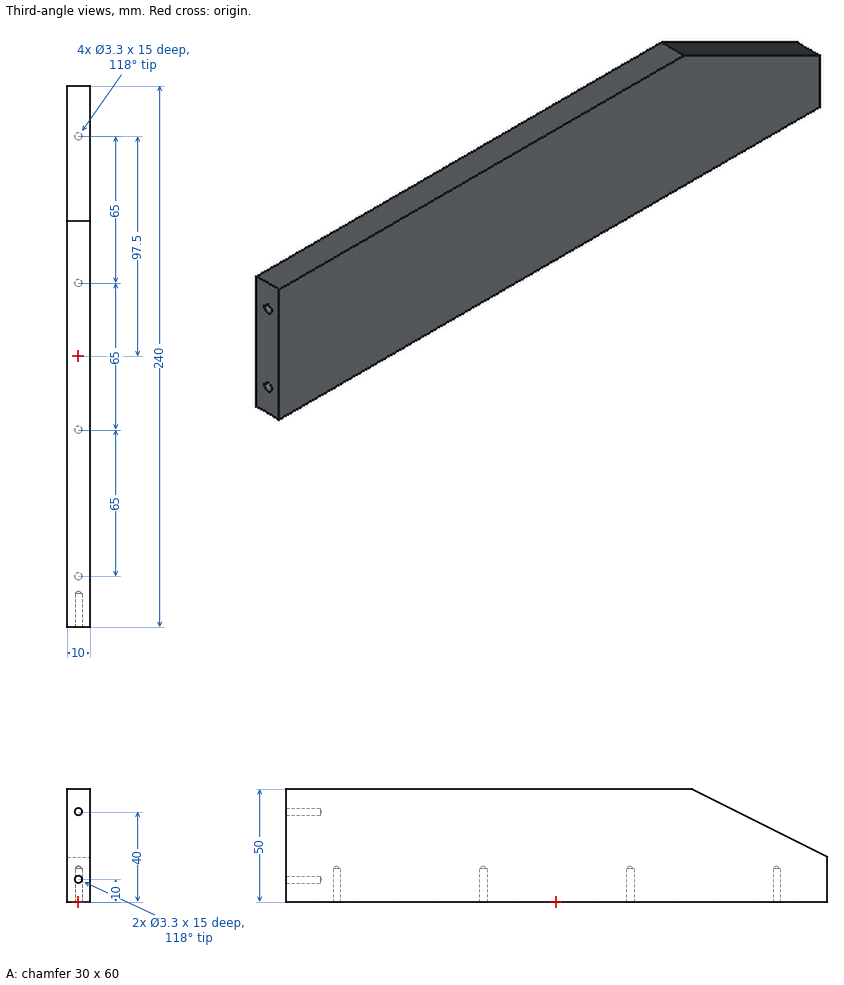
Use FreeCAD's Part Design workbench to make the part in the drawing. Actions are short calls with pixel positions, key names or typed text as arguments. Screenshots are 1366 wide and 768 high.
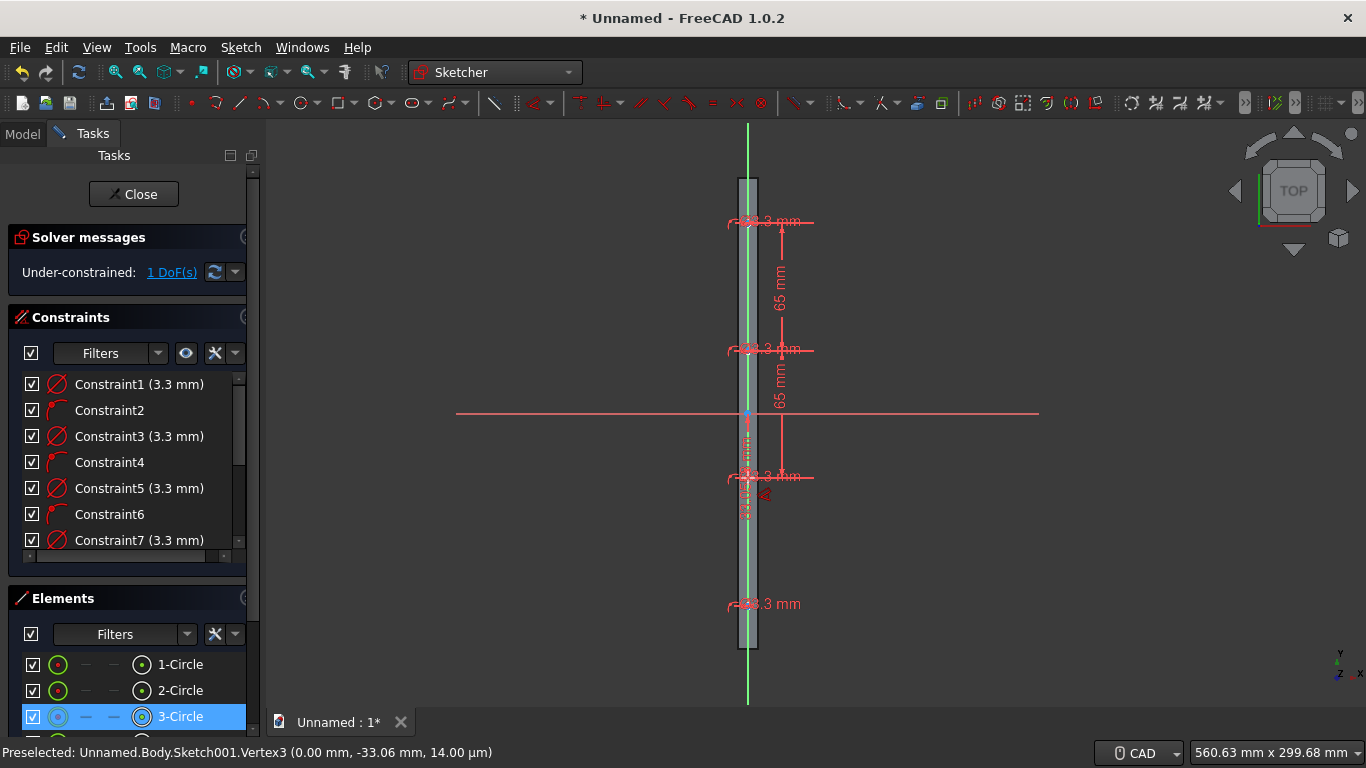
click(748, 606)
click(782, 542)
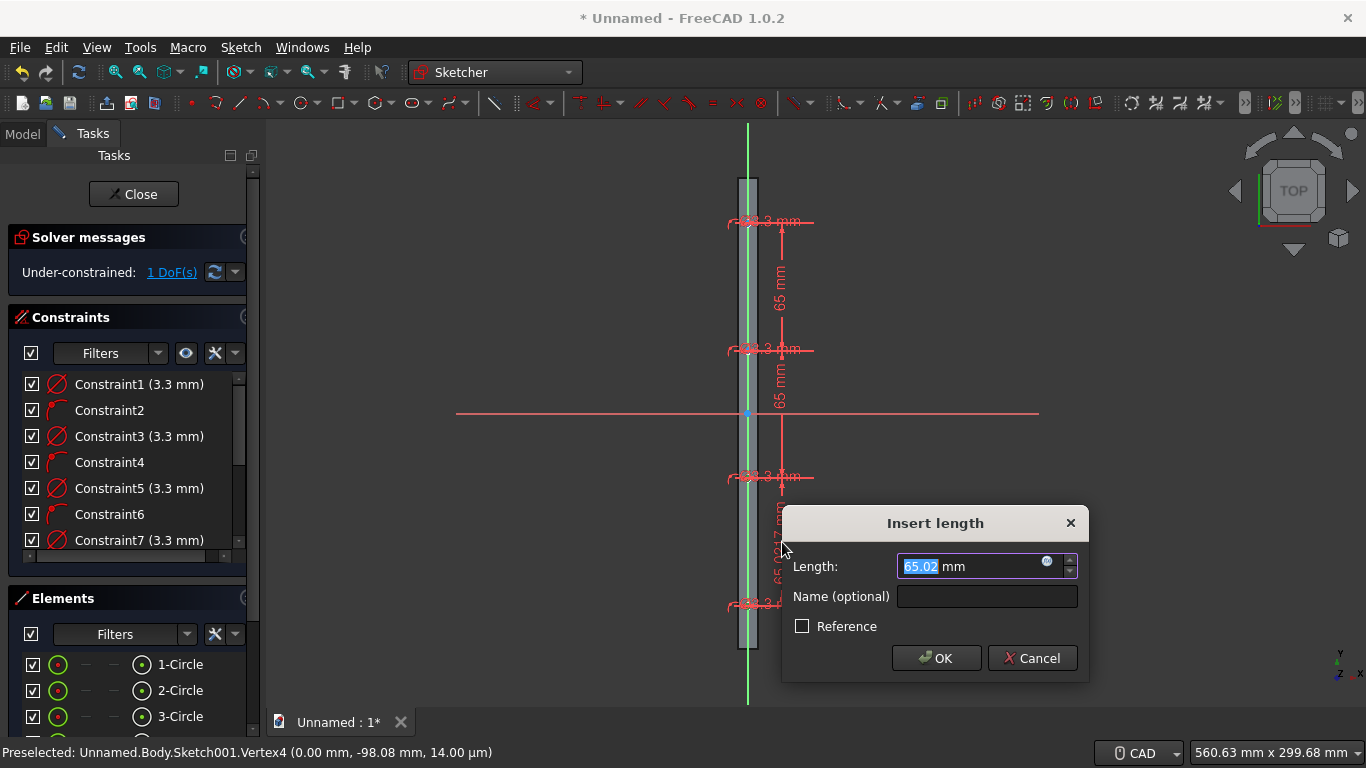
text(65)
key(Return)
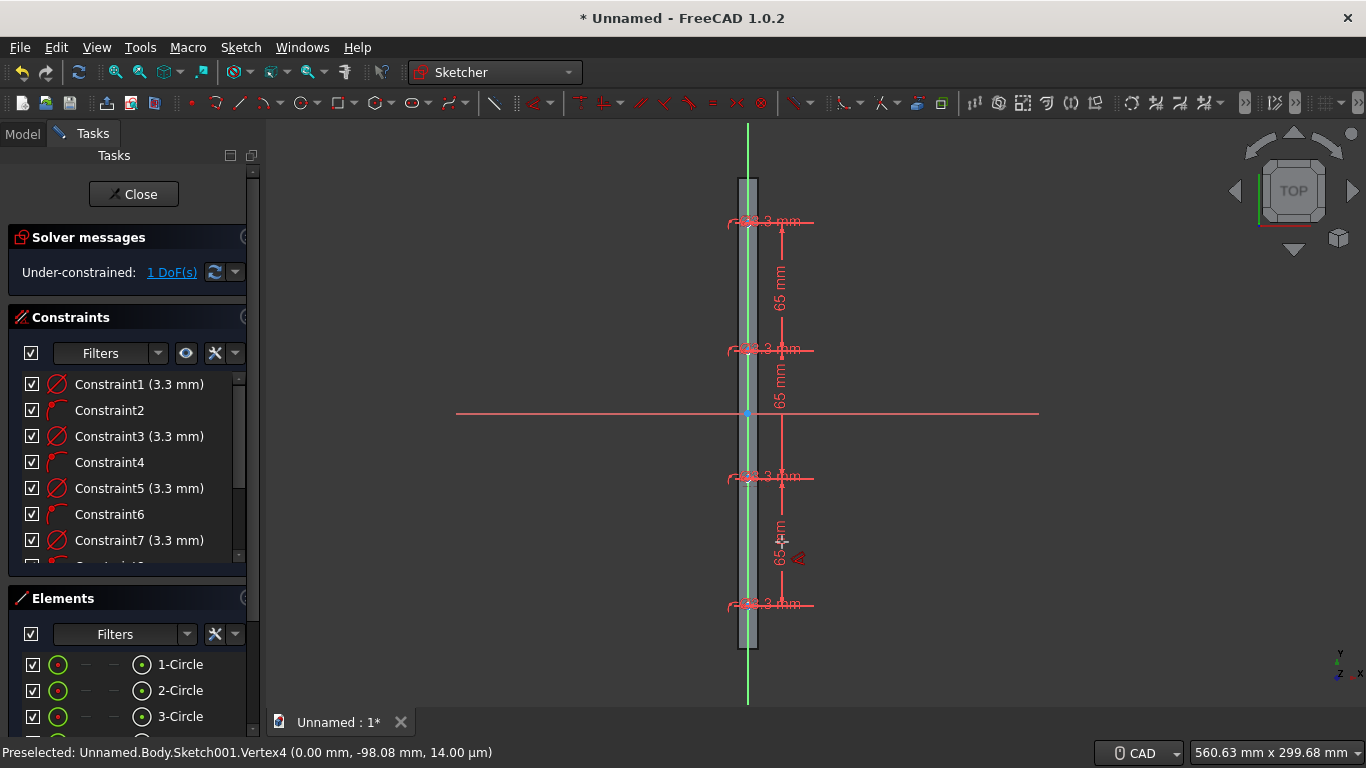
click(748, 223)
click(782, 319)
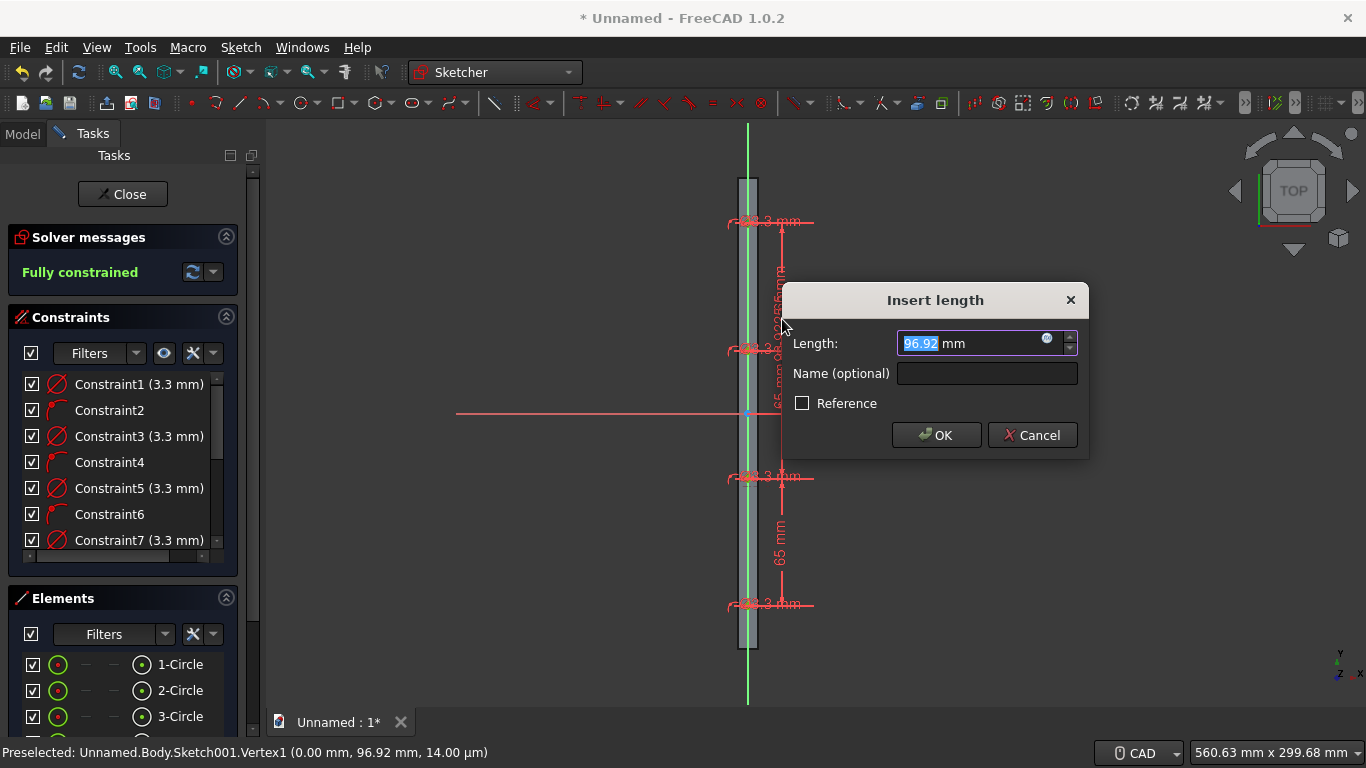
text(97.5)
key(Return)
key(Escape)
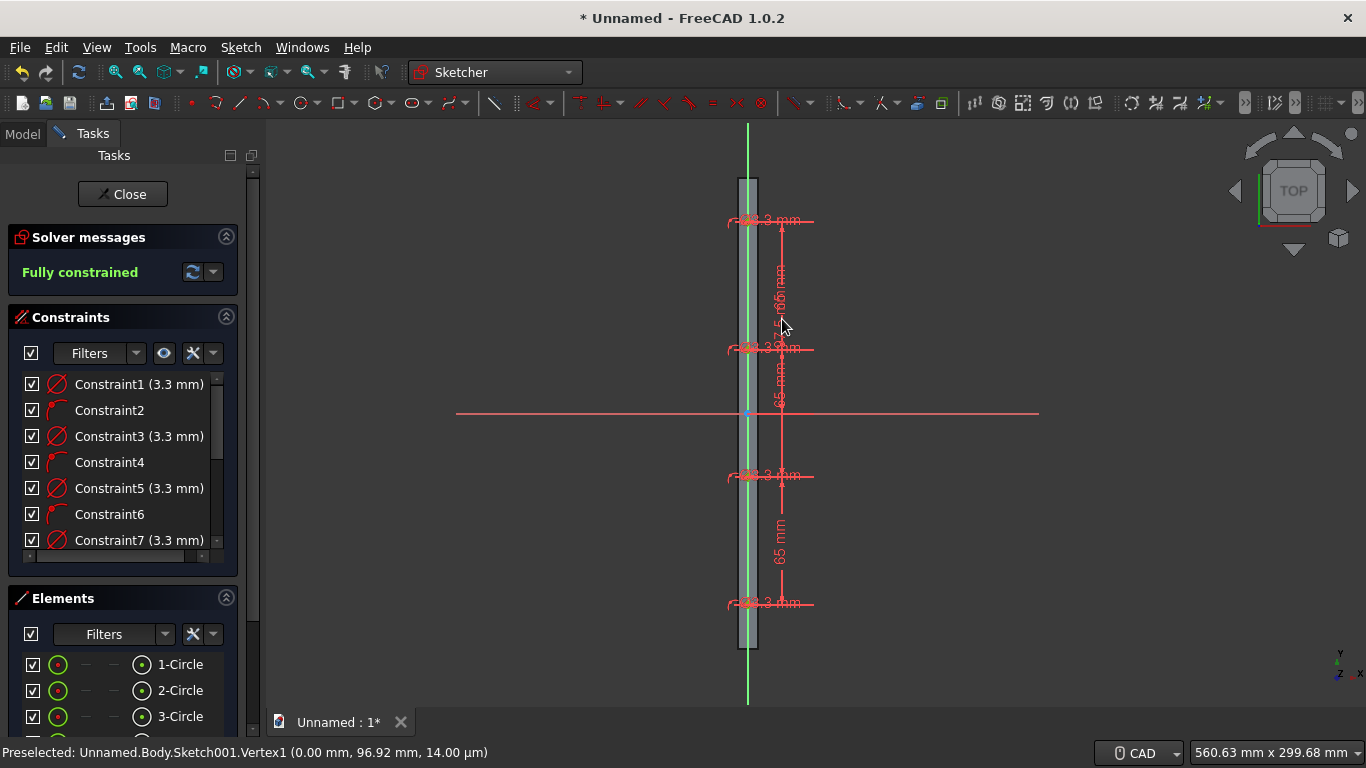
click(123, 194)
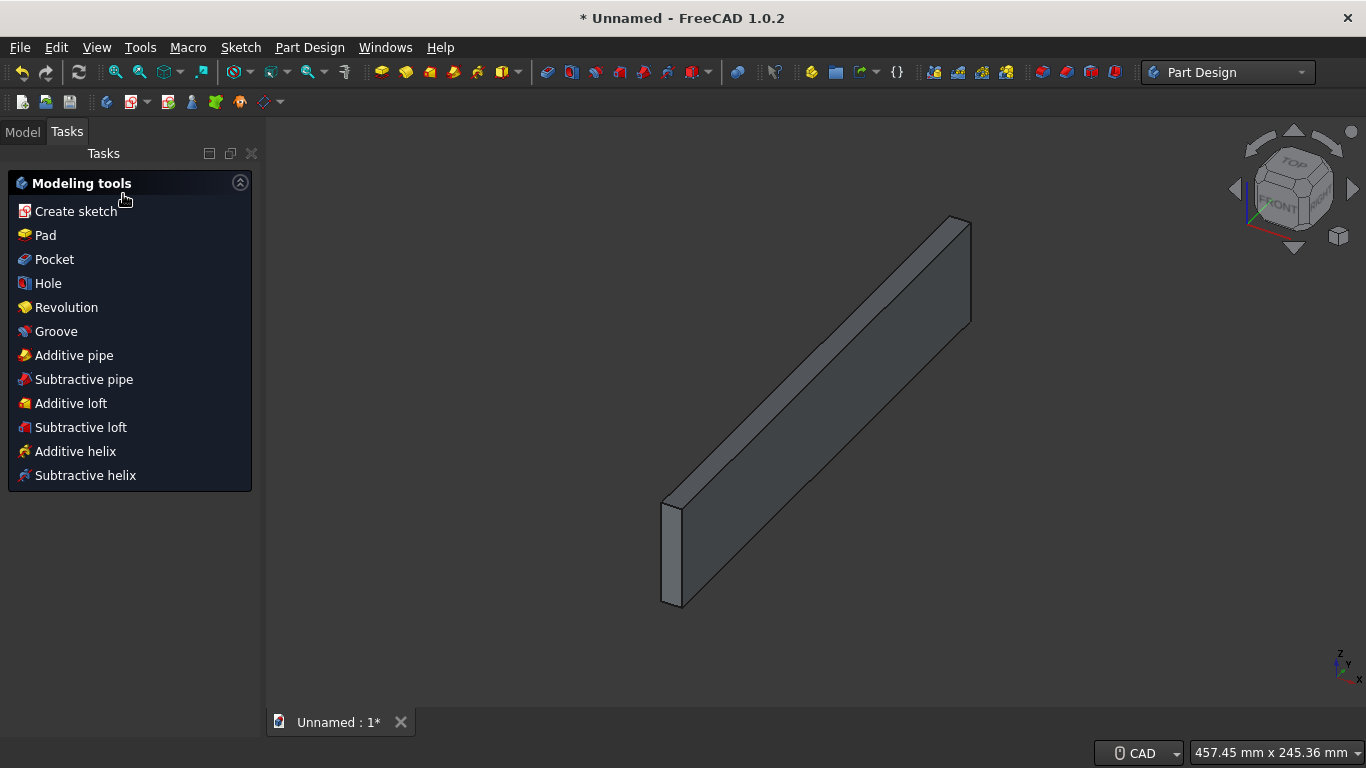
click(572, 72)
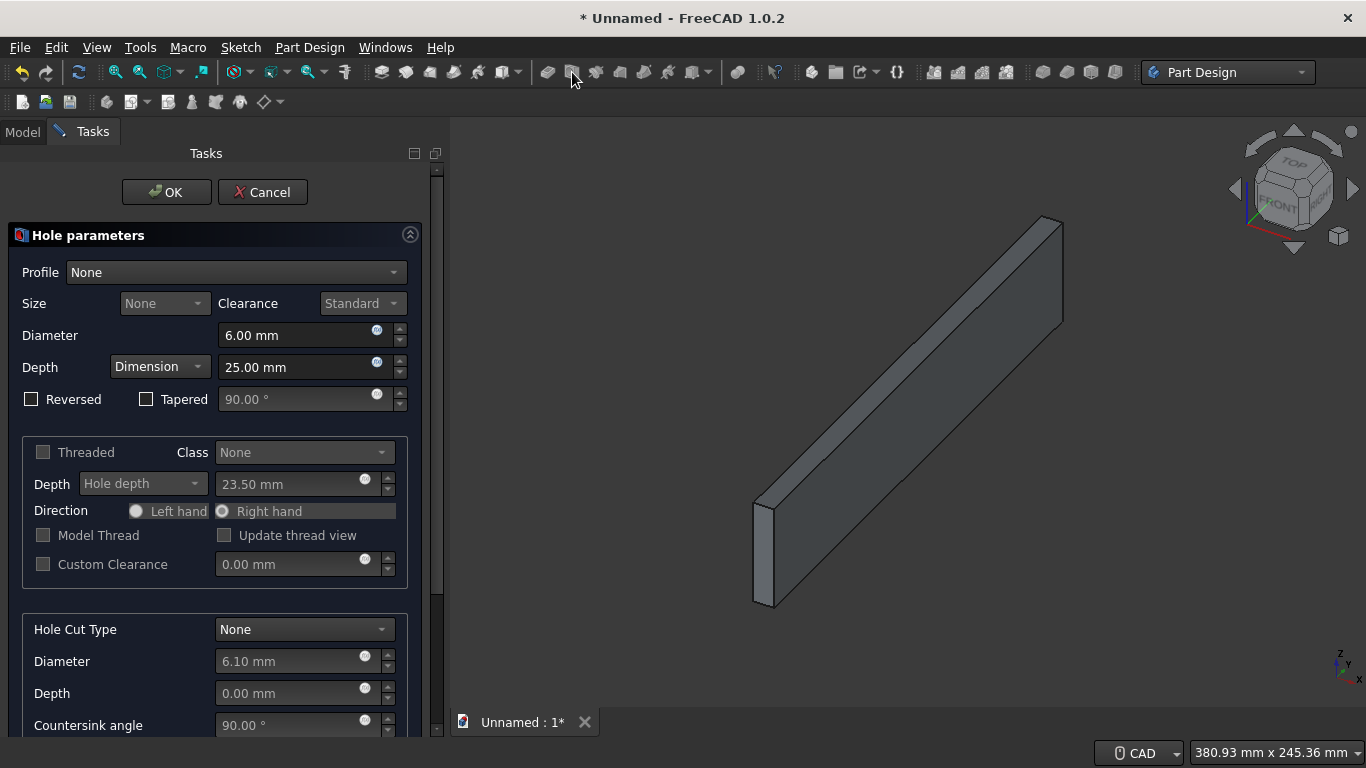
triple_click(305, 335)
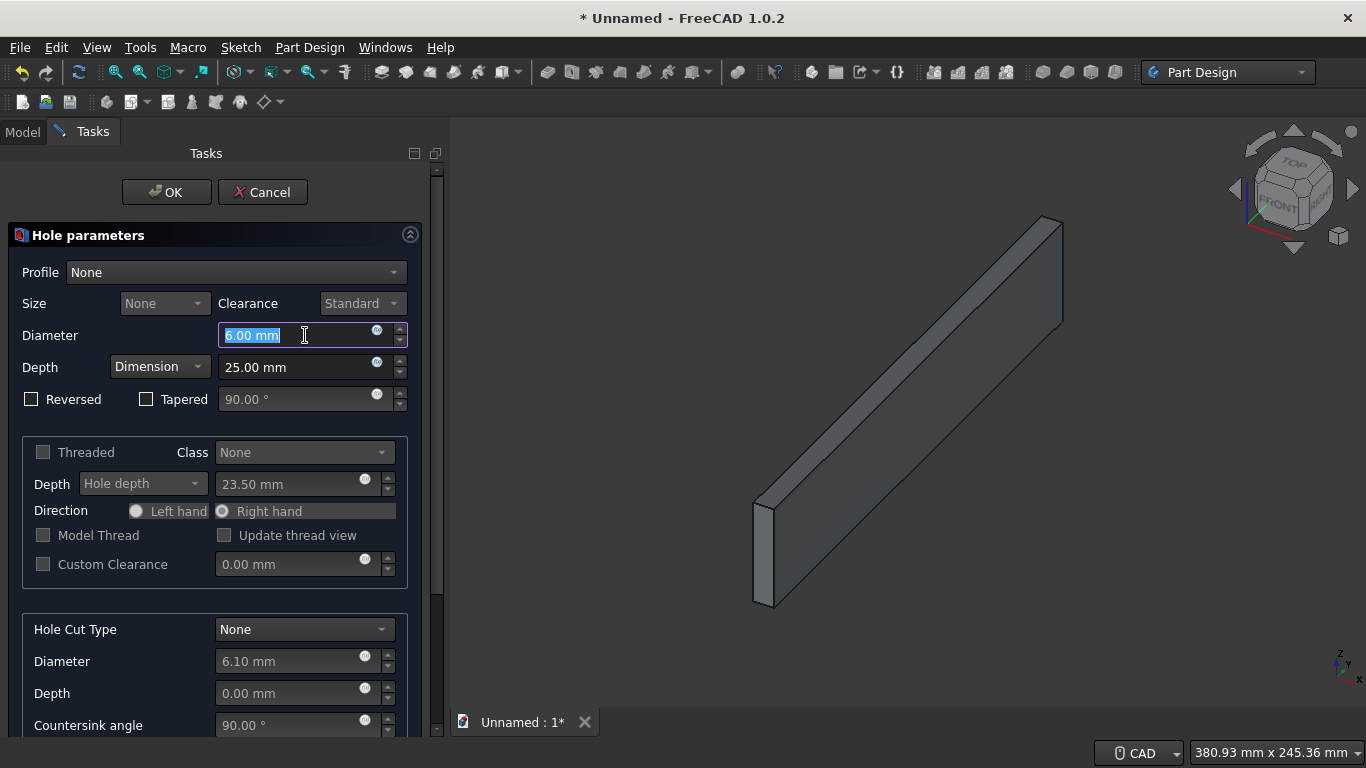
text(3.3)
key(Tab)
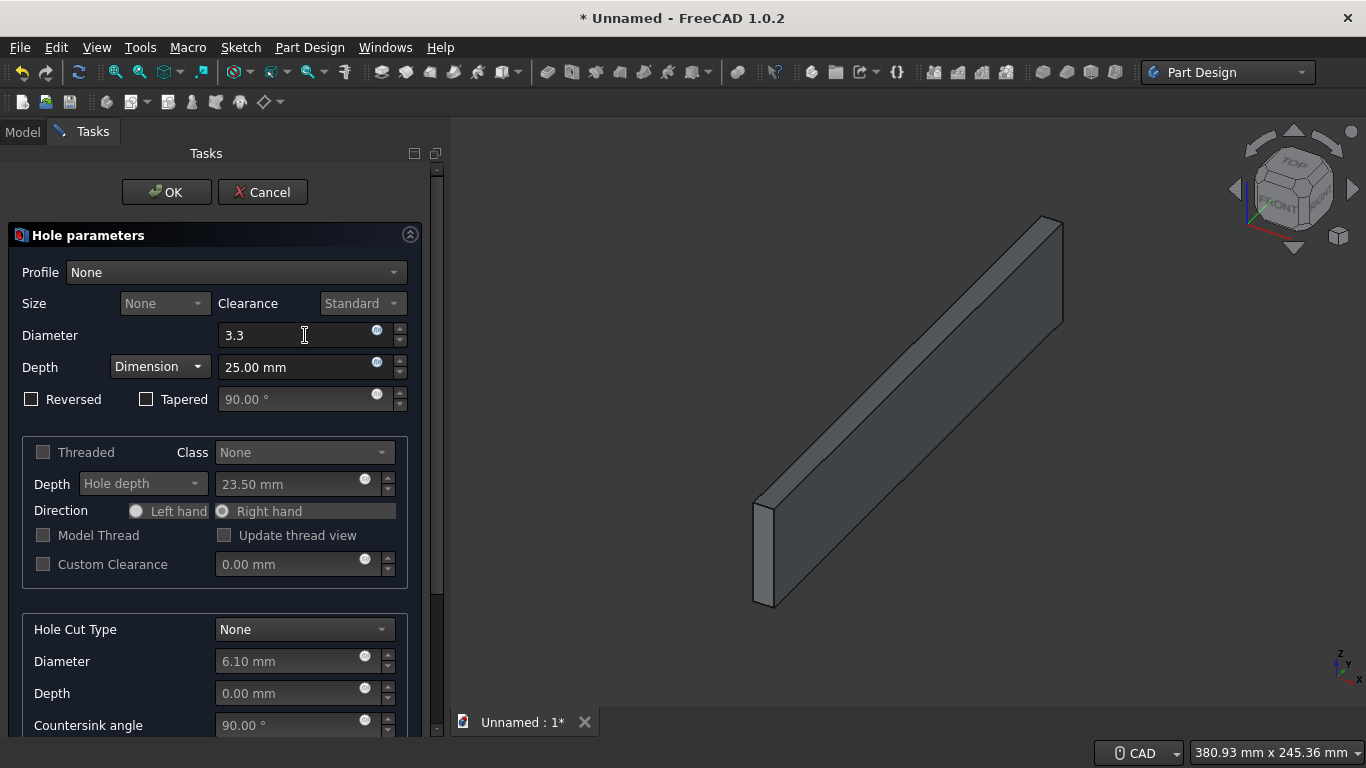
triple_click(305, 367)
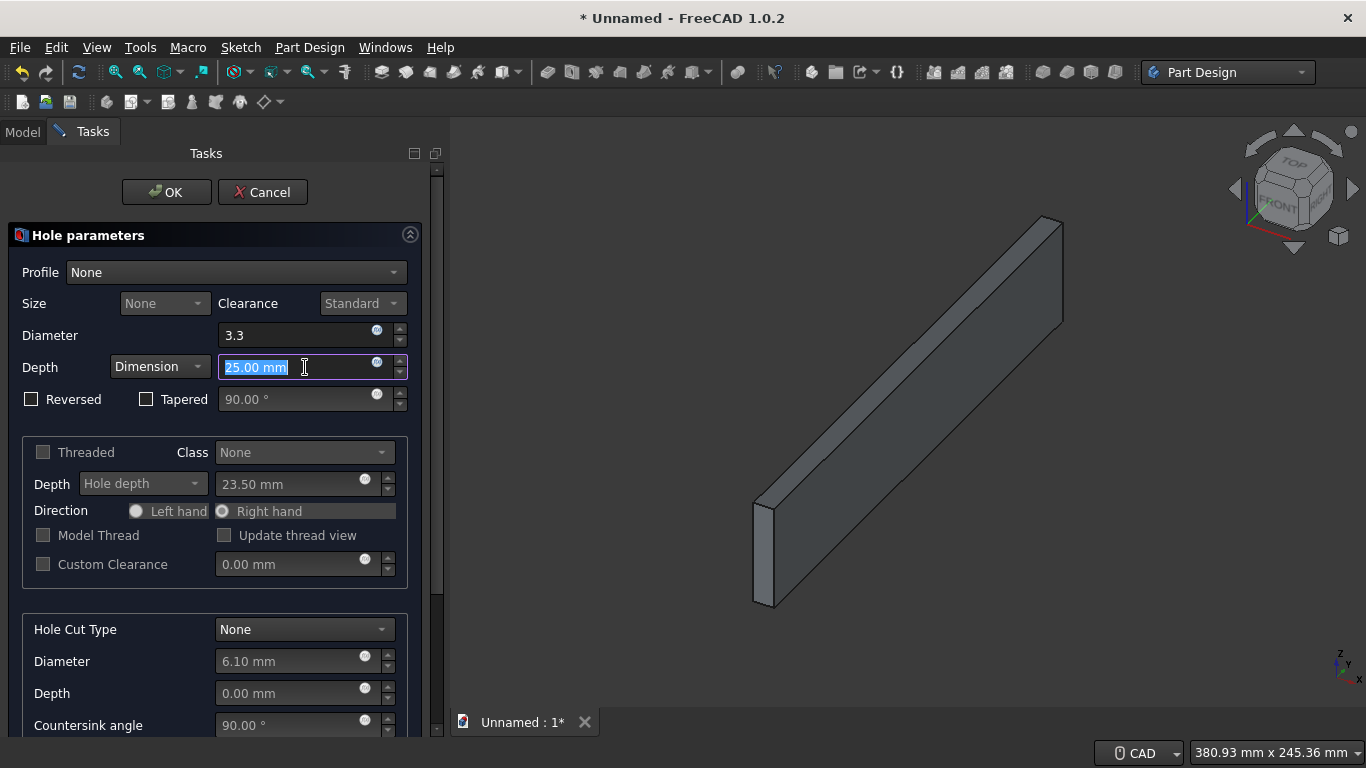
text(15)
key(Tab)